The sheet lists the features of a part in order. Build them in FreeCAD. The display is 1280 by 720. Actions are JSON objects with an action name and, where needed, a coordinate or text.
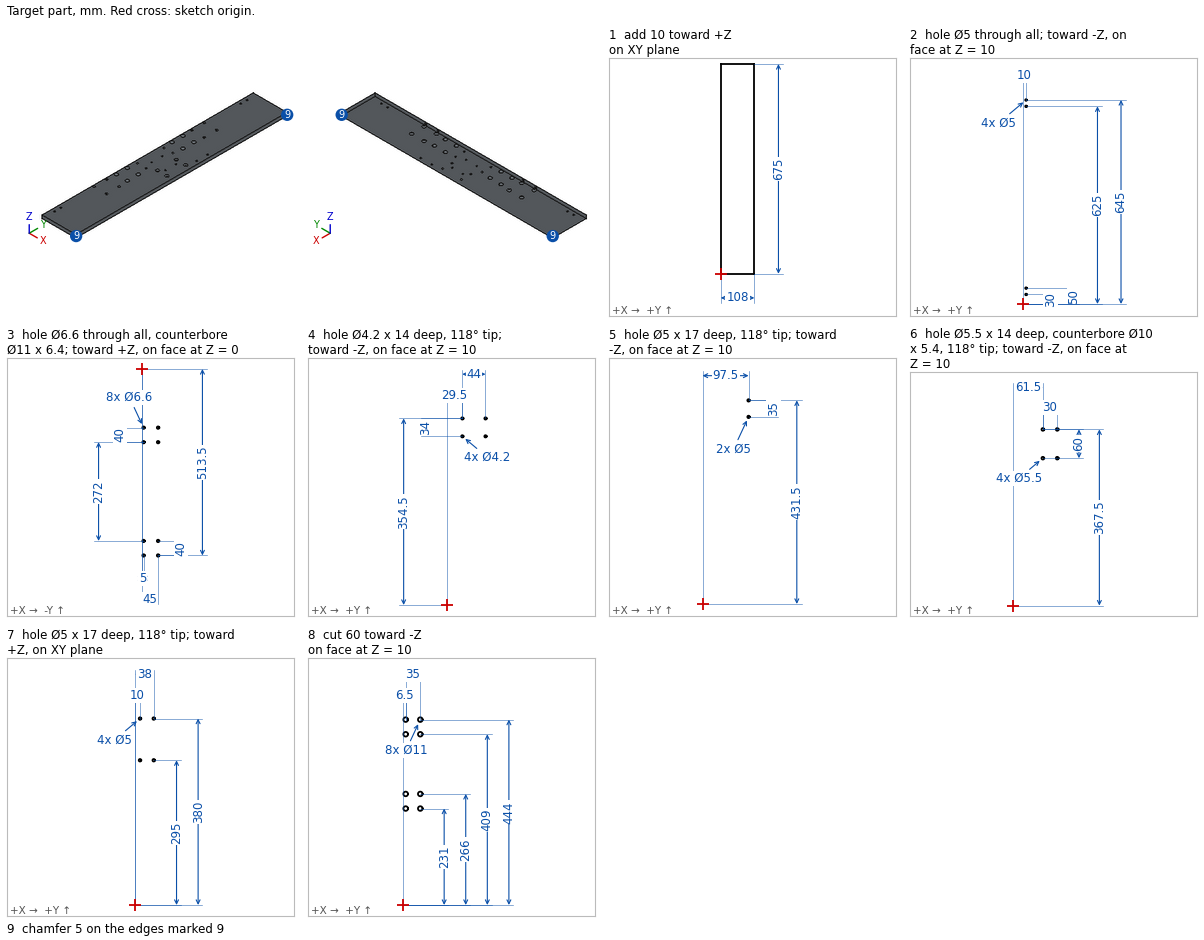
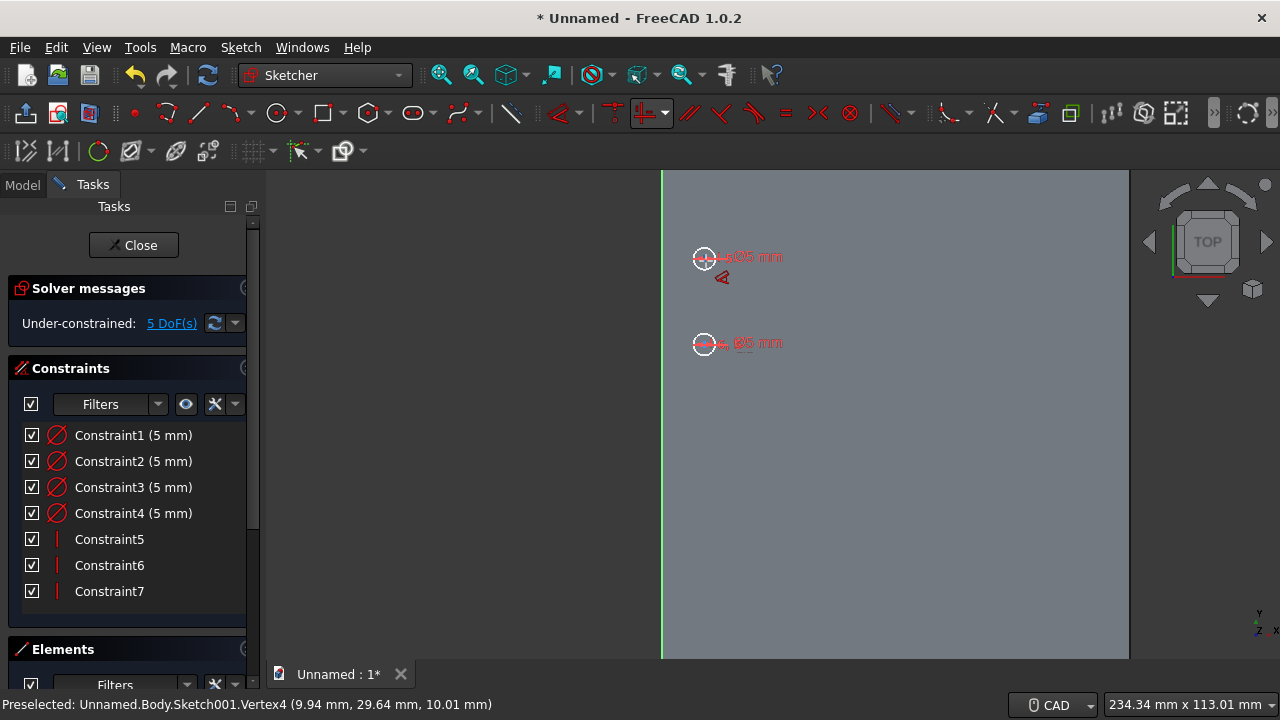
{"action": "left_click", "coordinate": [704, 259]}
{"action": "left_click", "coordinate": [683, 225]}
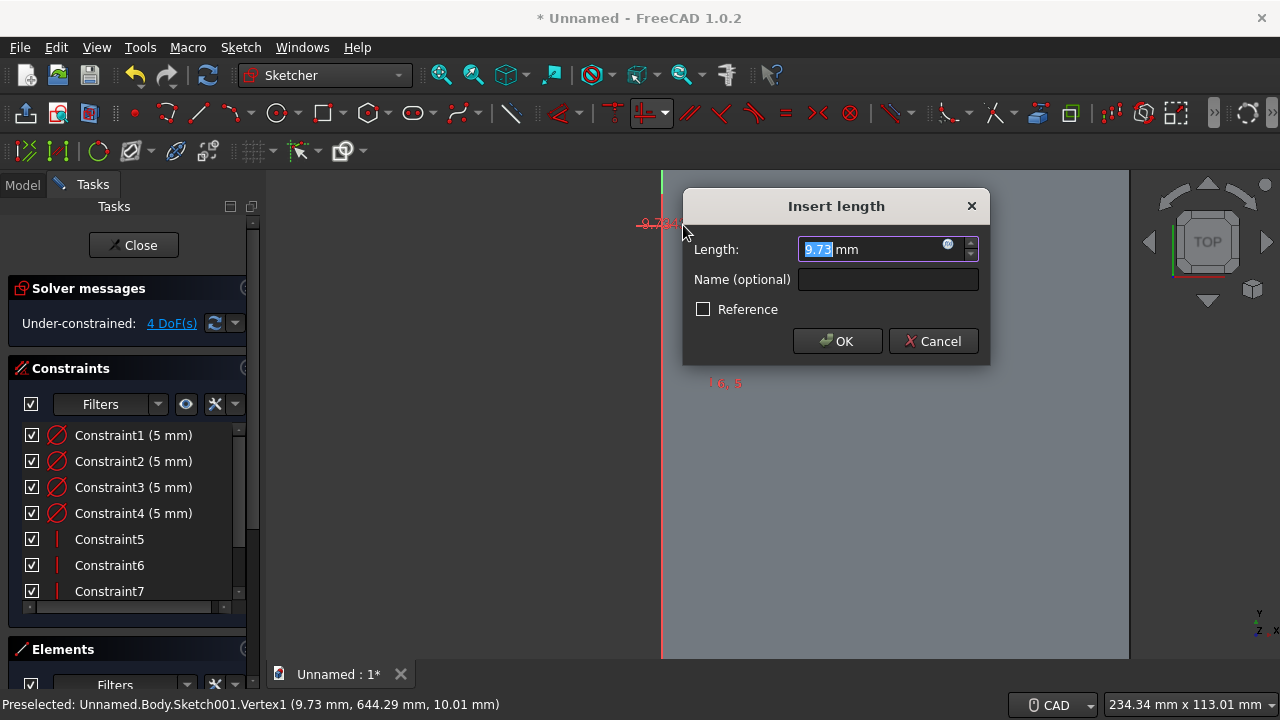
{"action": "type", "text": "10"}
{"action": "key", "text": "Return"}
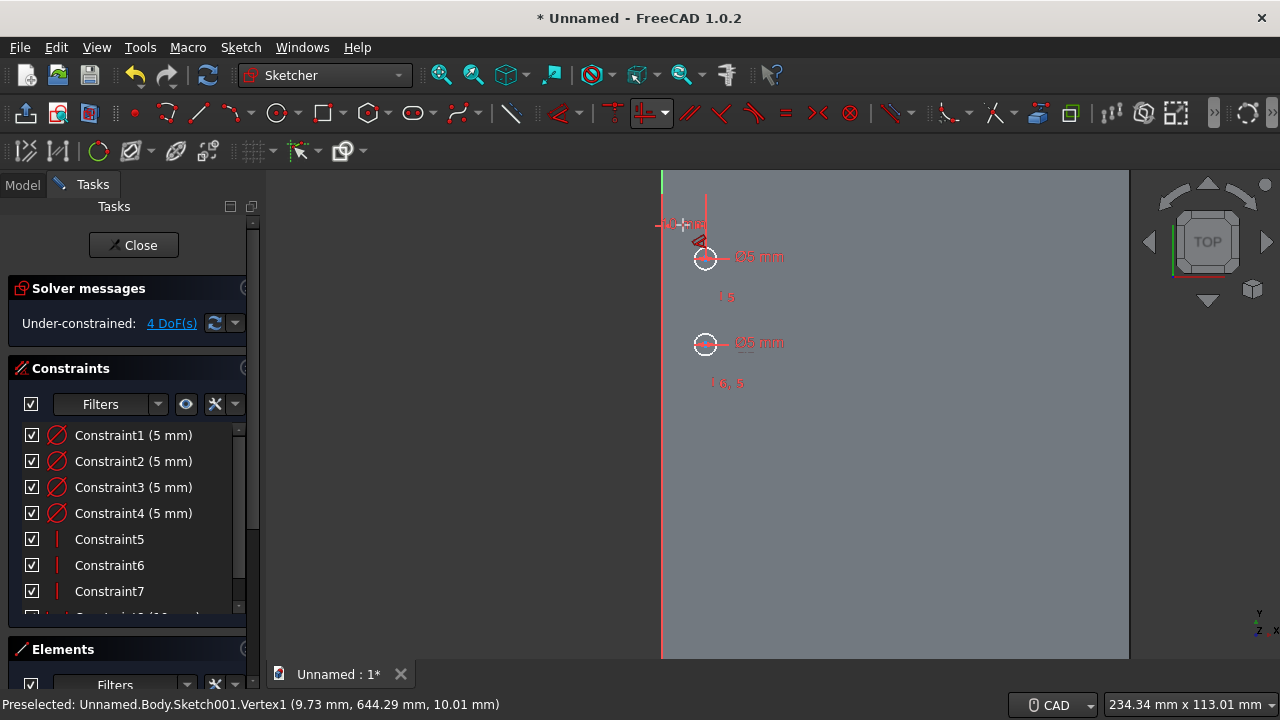
{"action": "scroll", "coordinate": [706, 261], "scroll_direction": "down", "scroll_amount": 11}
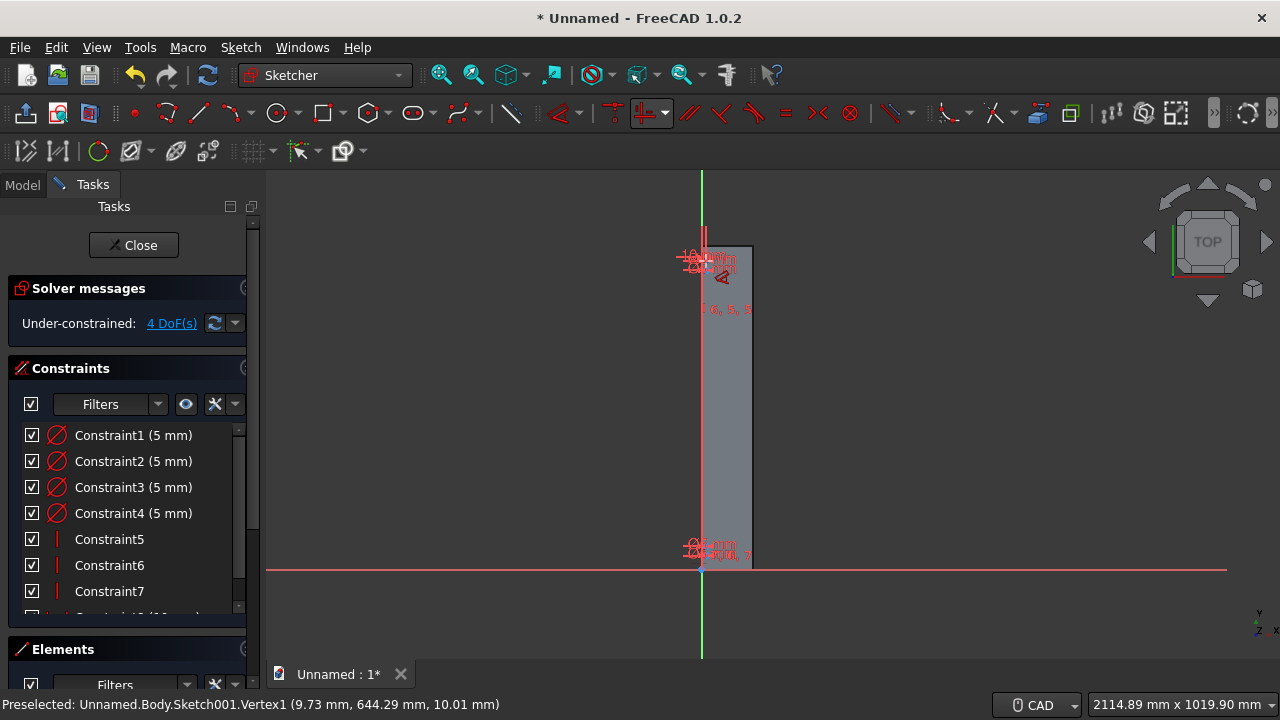
{"action": "scroll", "coordinate": [706, 546], "scroll_direction": "up", "scroll_amount": 3}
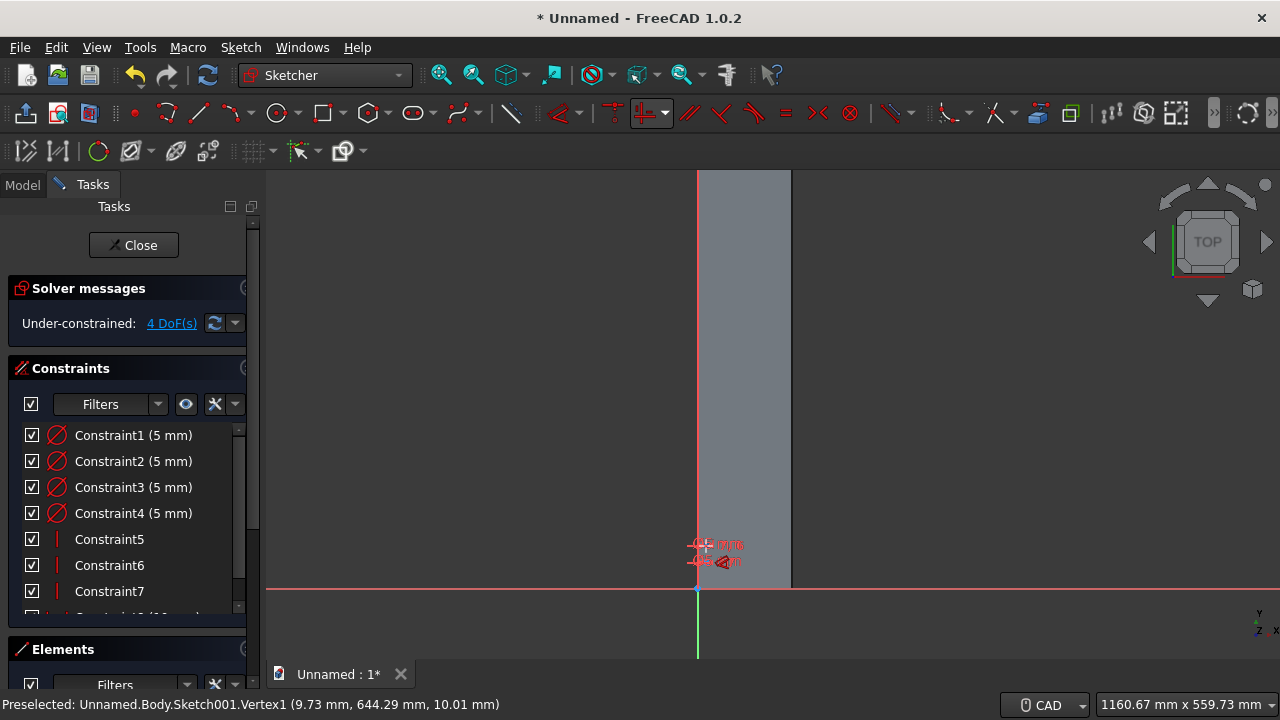
{"action": "left_click", "coordinate": [706, 546]}
{"action": "left_click", "coordinate": [664, 567]}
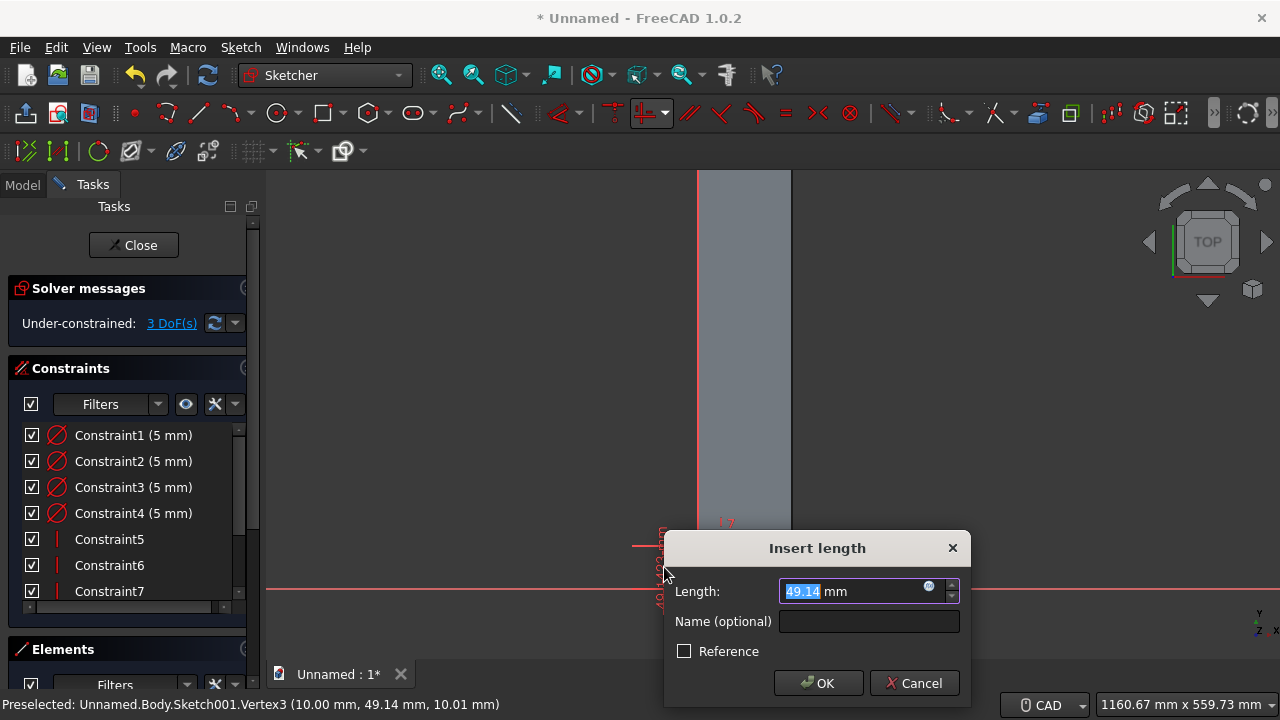
{"action": "type", "text": "50"}
{"action": "key", "text": "Return"}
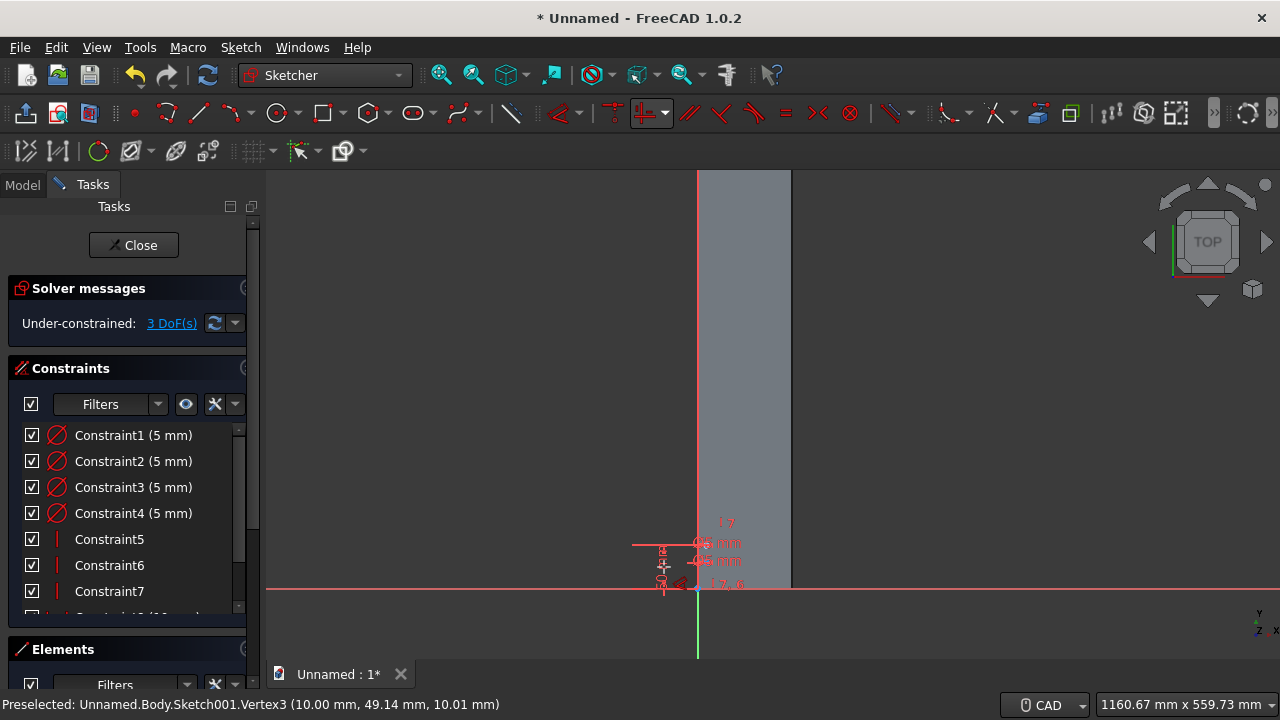
{"action": "scroll", "coordinate": [706, 563], "scroll_direction": "up", "scroll_amount": 3}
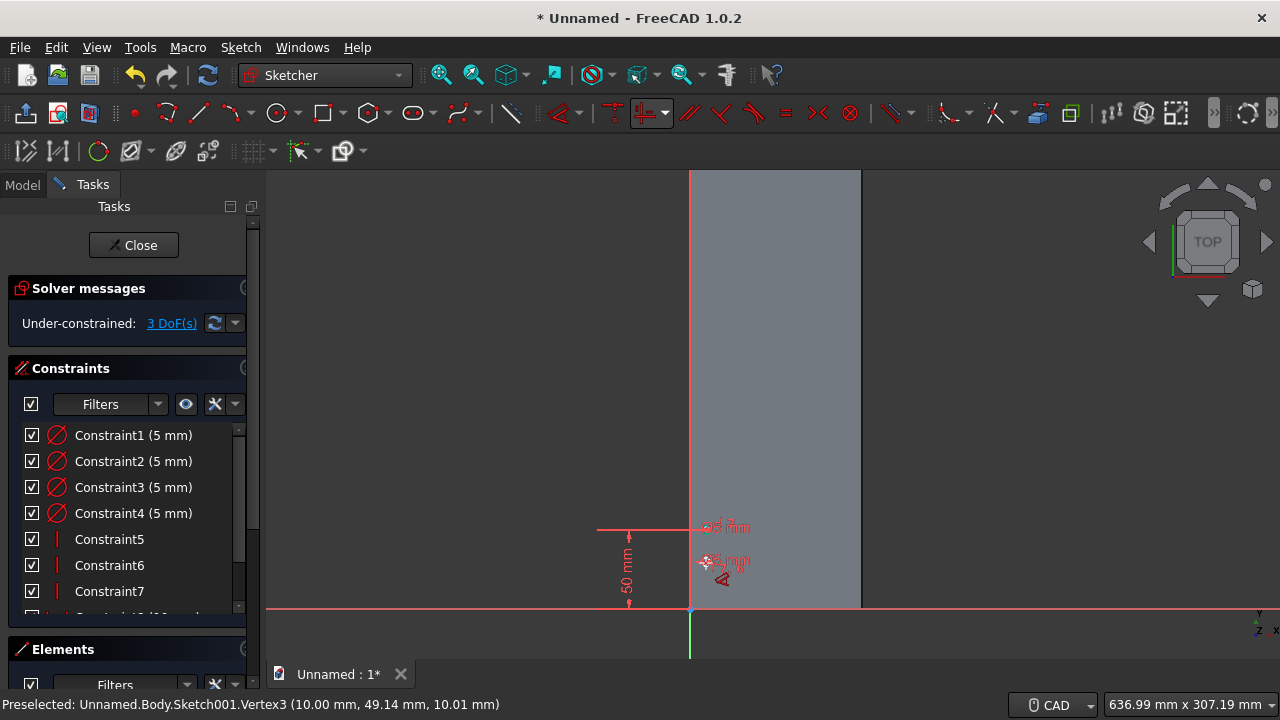
{"action": "left_click", "coordinate": [706, 562]}
{"action": "left_click", "coordinate": [740, 586]}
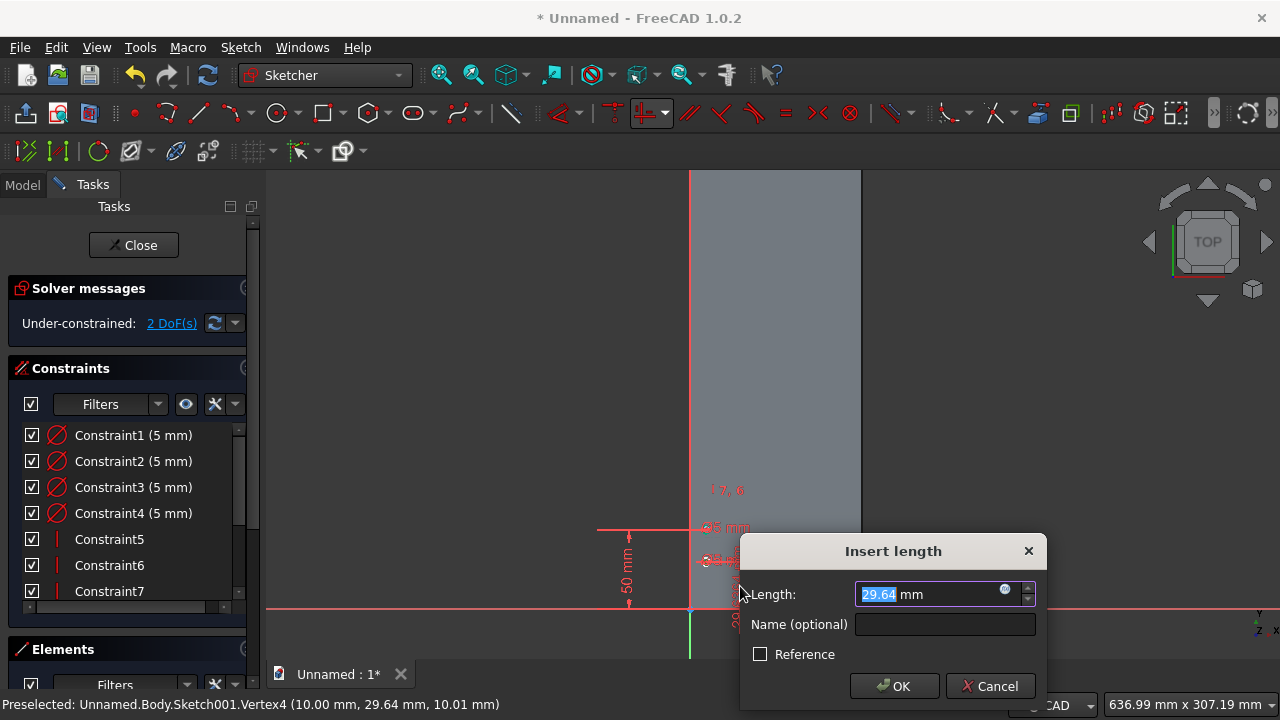
{"action": "type", "text": "30"}
{"action": "key", "text": "Return"}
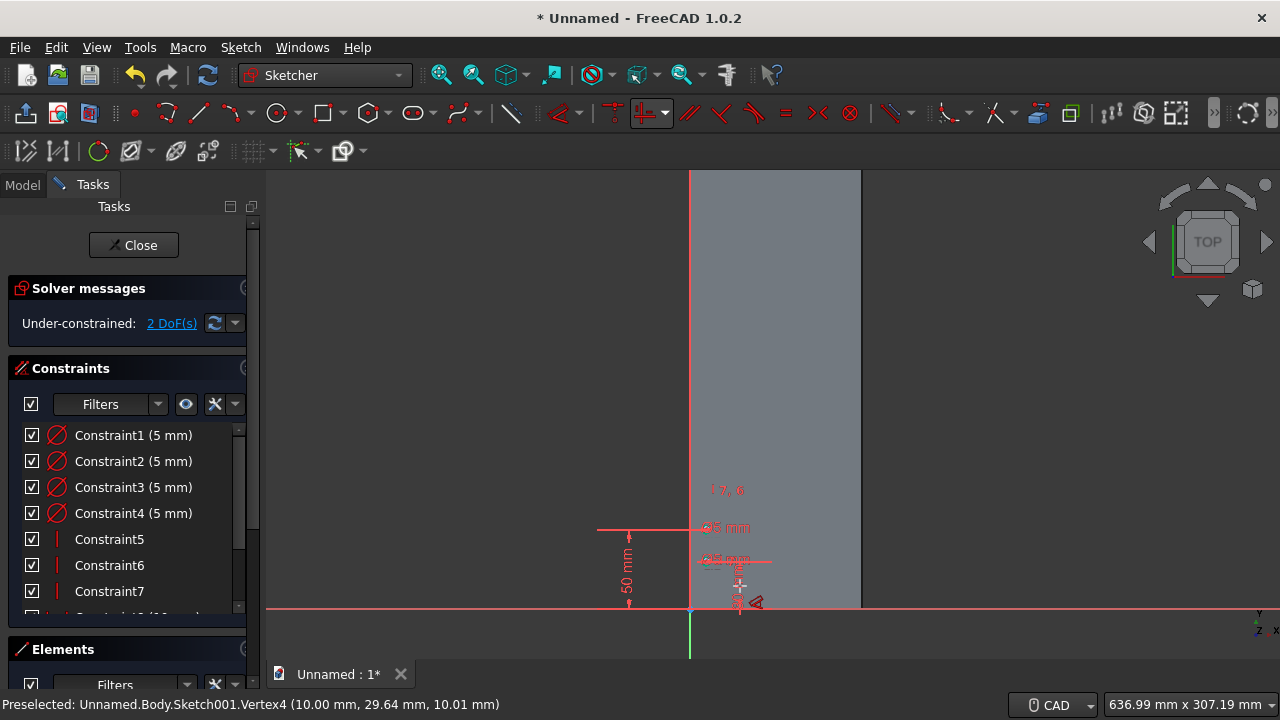
{"action": "scroll", "coordinate": [706, 553], "scroll_direction": "down", "scroll_amount": 6}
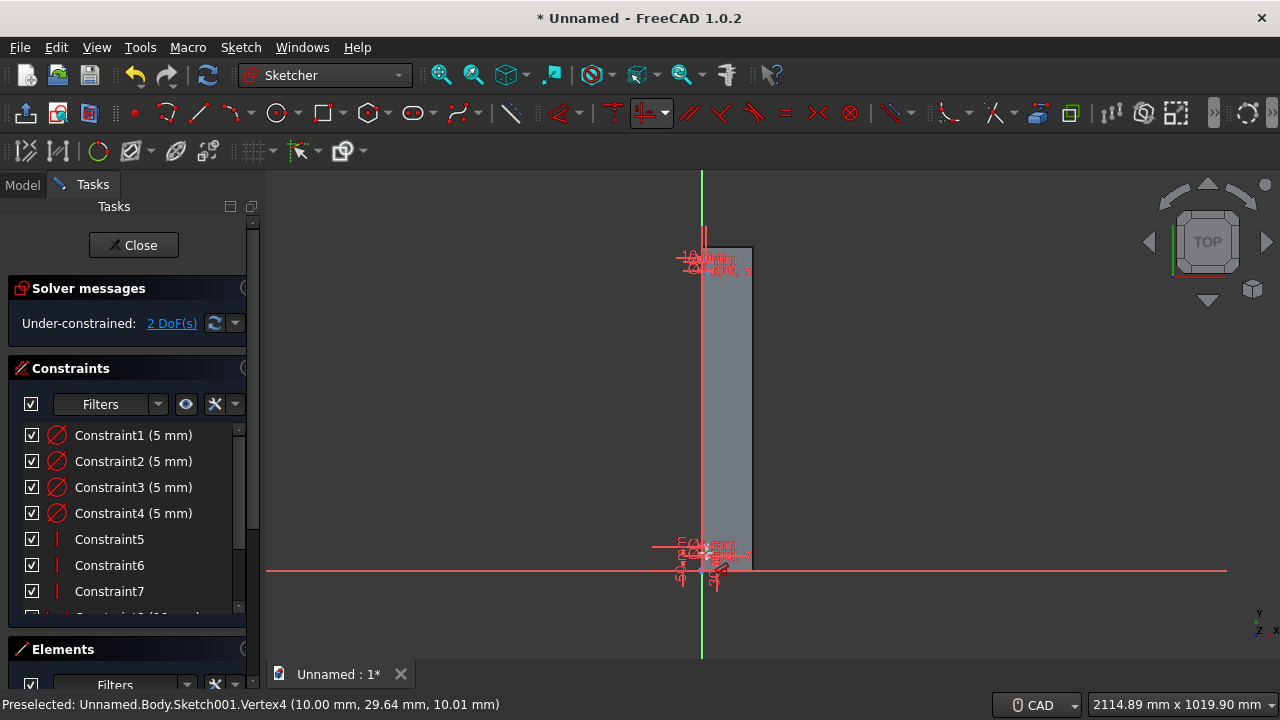
{"action": "scroll", "coordinate": [706, 262], "scroll_direction": "up", "scroll_amount": 2}